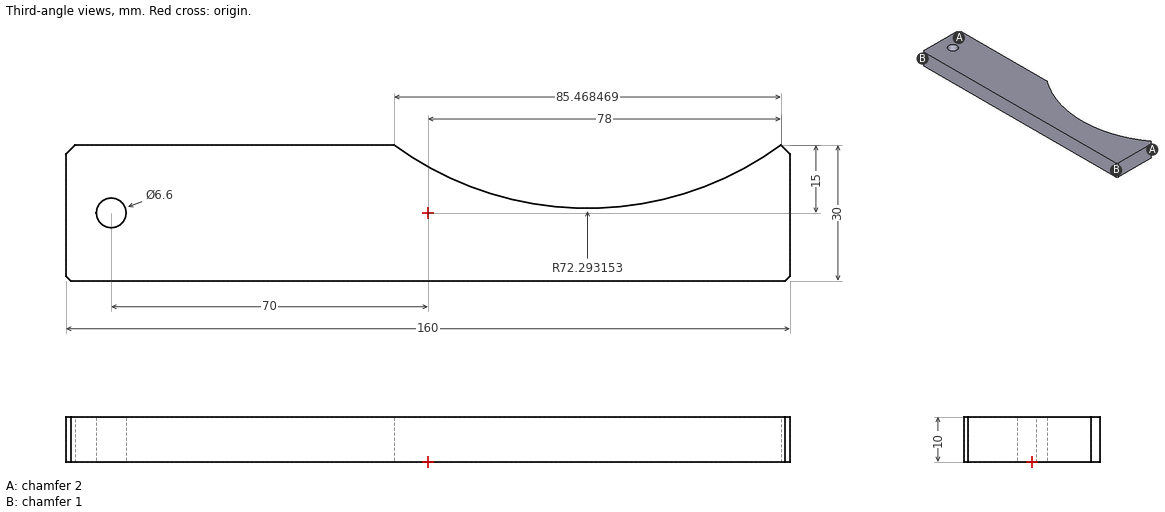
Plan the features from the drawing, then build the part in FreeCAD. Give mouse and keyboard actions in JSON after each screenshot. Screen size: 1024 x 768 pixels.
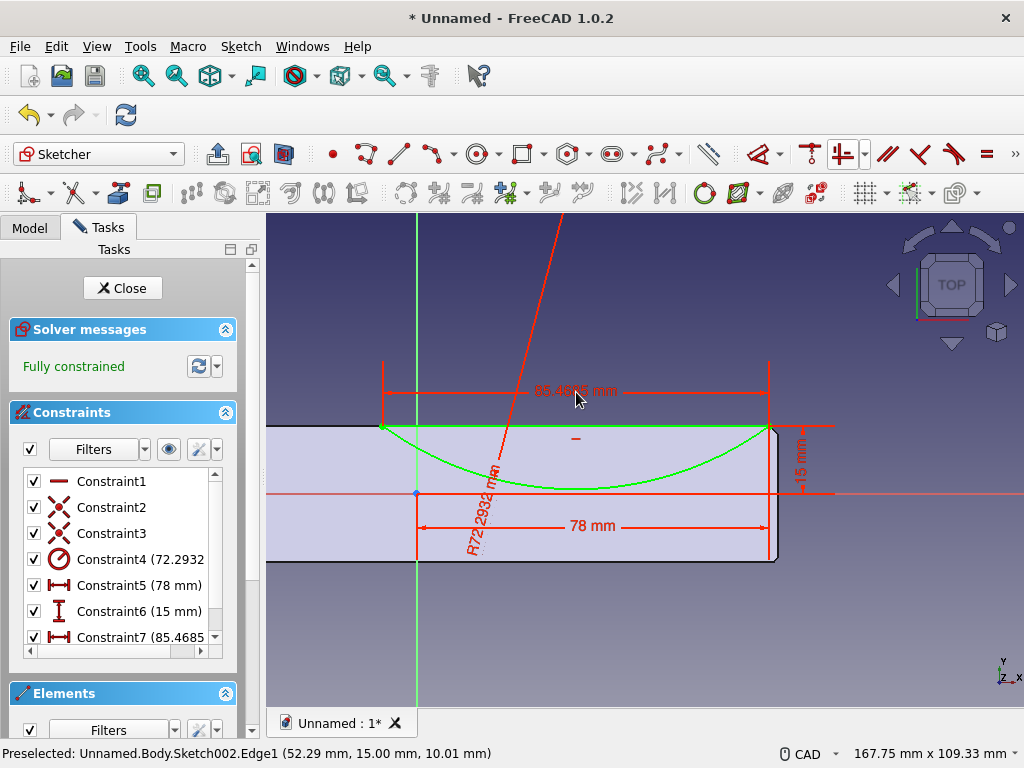
{"action": "left_click", "coordinate": [123, 288]}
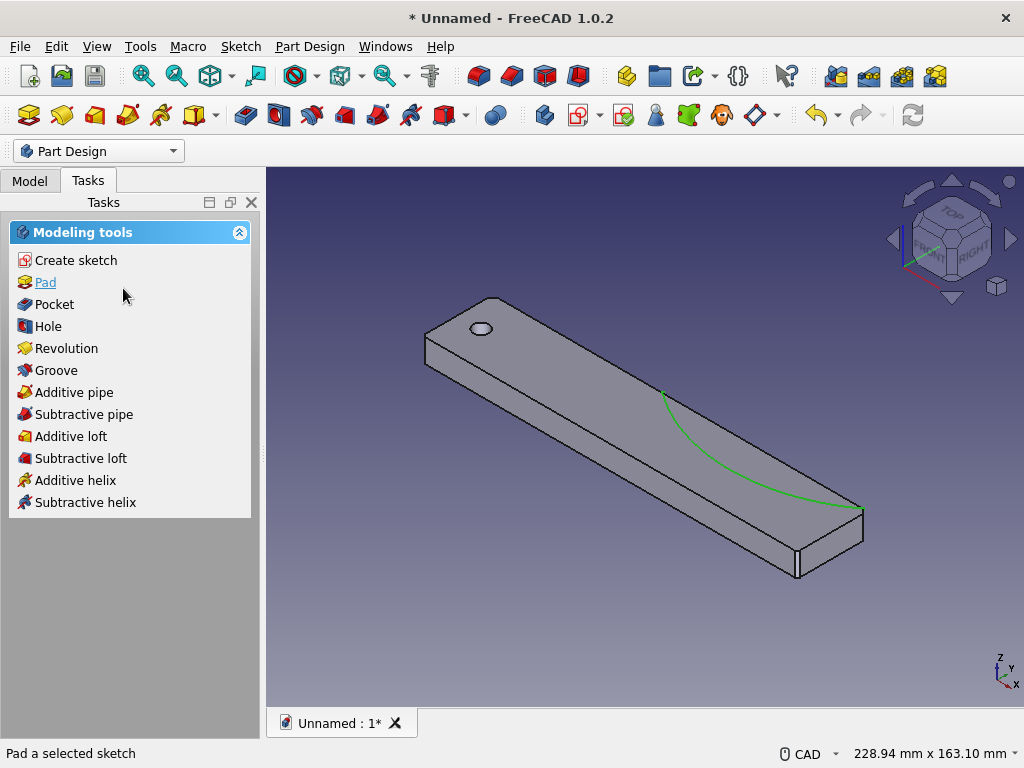
{"action": "left_click", "coordinate": [246, 116]}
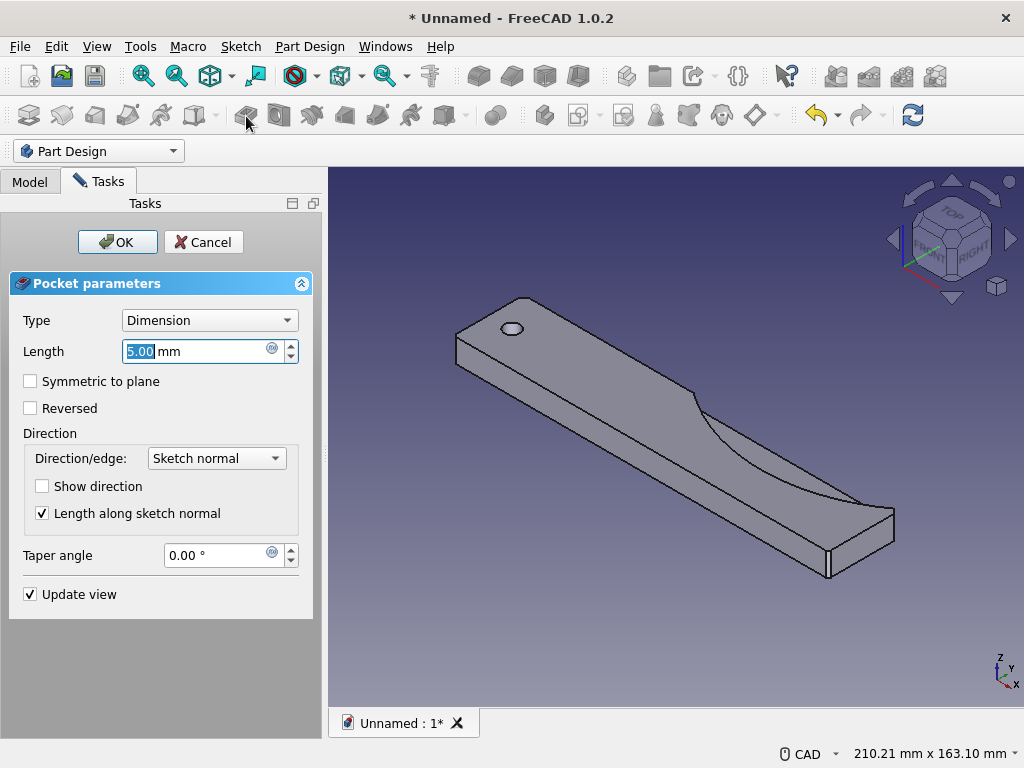
{"action": "left_click", "coordinate": [210, 320]}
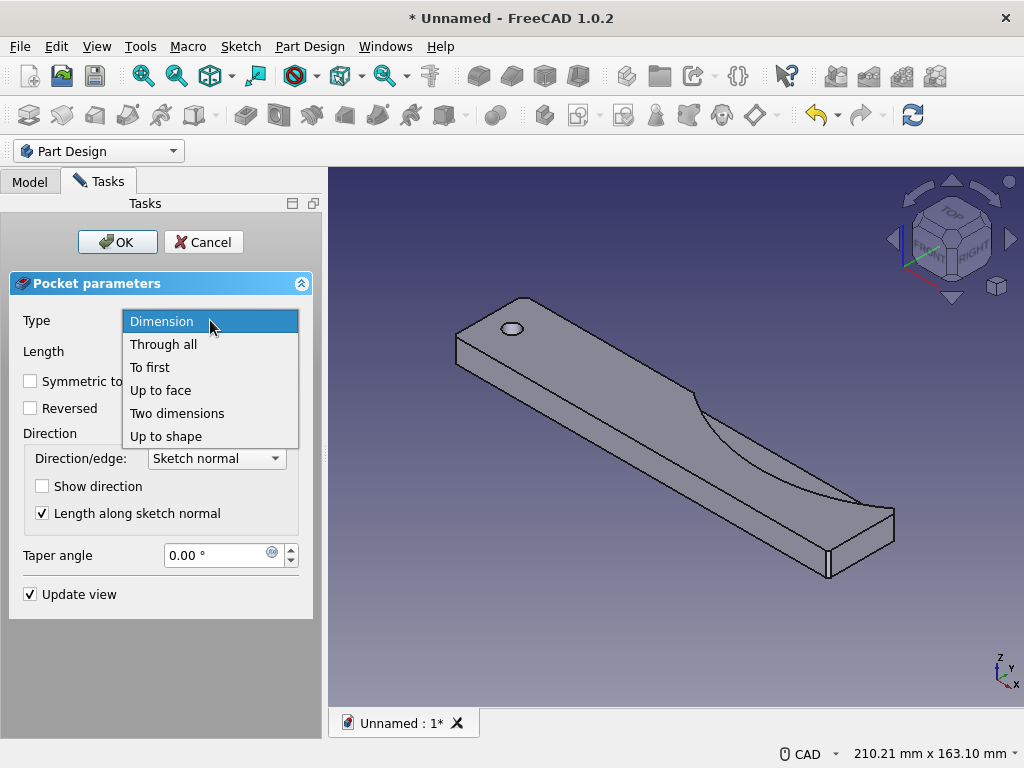
{"action": "left_click", "coordinate": [208, 344]}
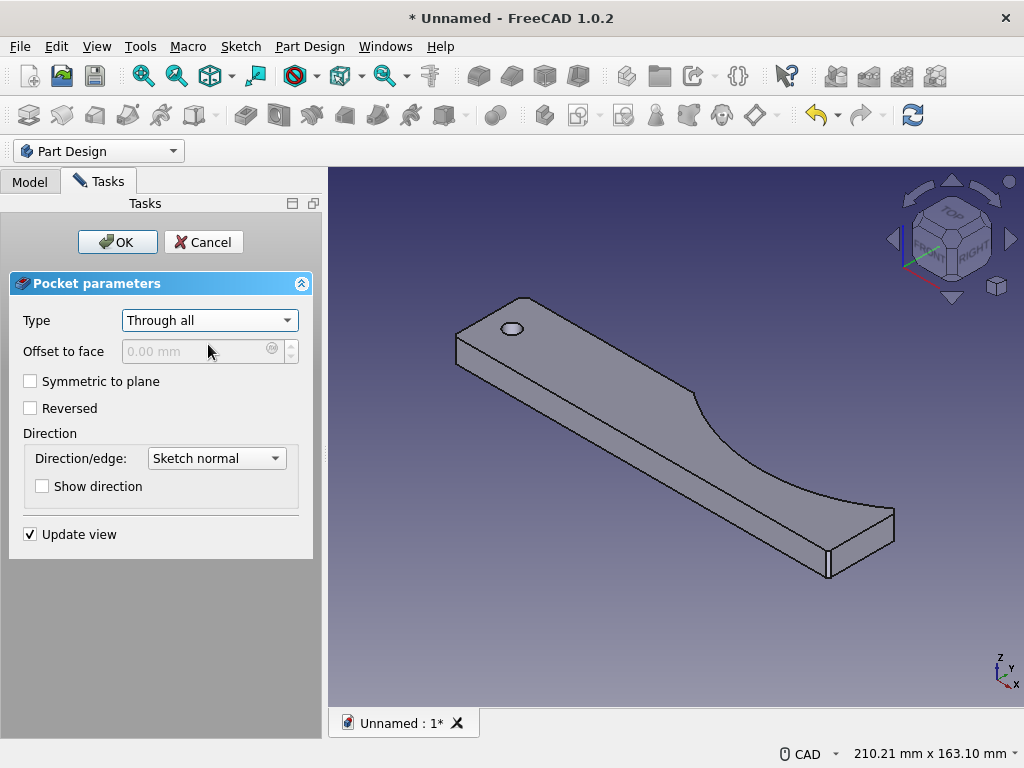
{"action": "left_click", "coordinate": [118, 242]}